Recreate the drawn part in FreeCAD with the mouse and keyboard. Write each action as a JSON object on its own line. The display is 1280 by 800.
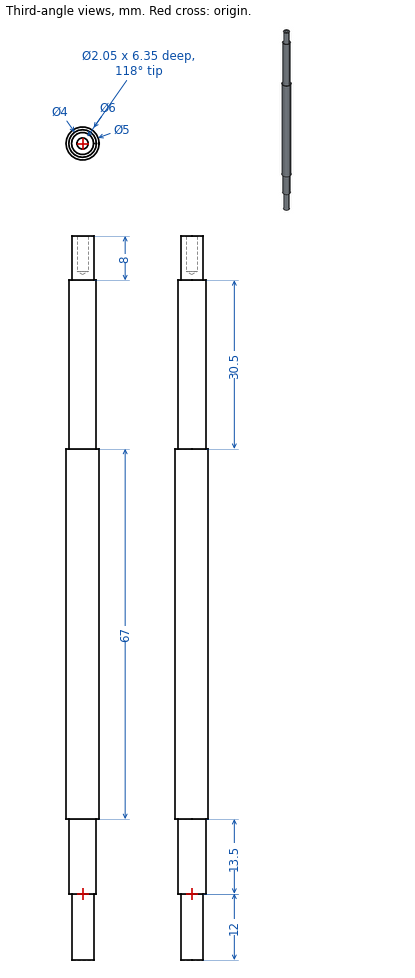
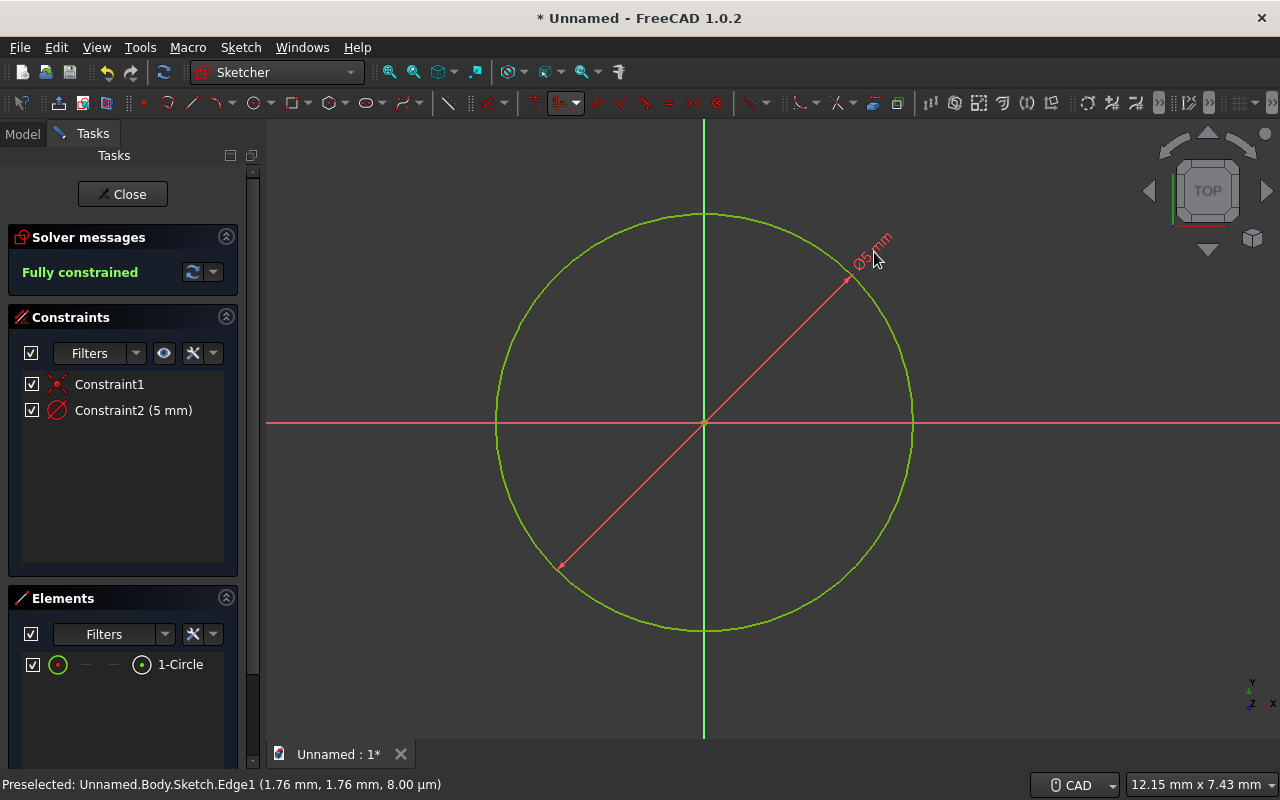
{"action": "left_click", "coordinate": [123, 194]}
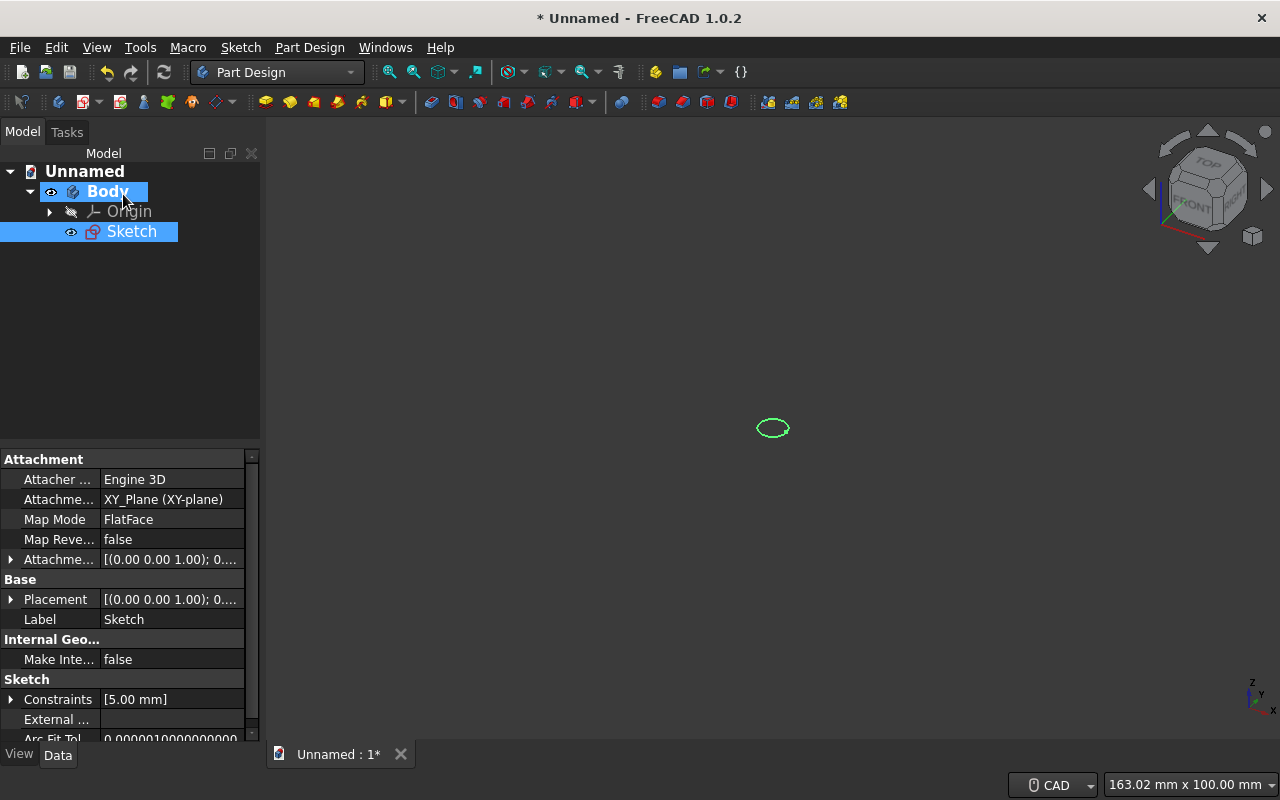
{"action": "left_click", "coordinate": [266, 102]}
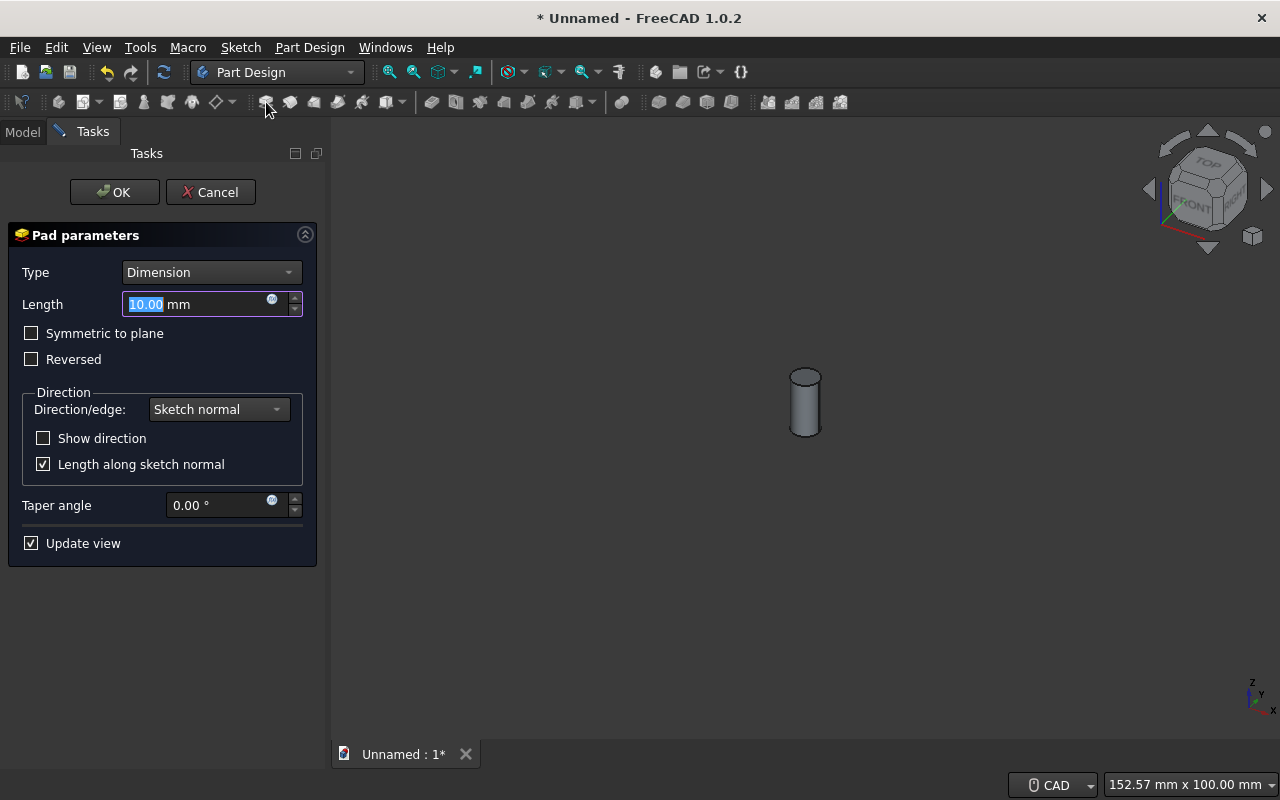
{"action": "type", "text": "13.5"}
{"action": "key", "text": "Tab"}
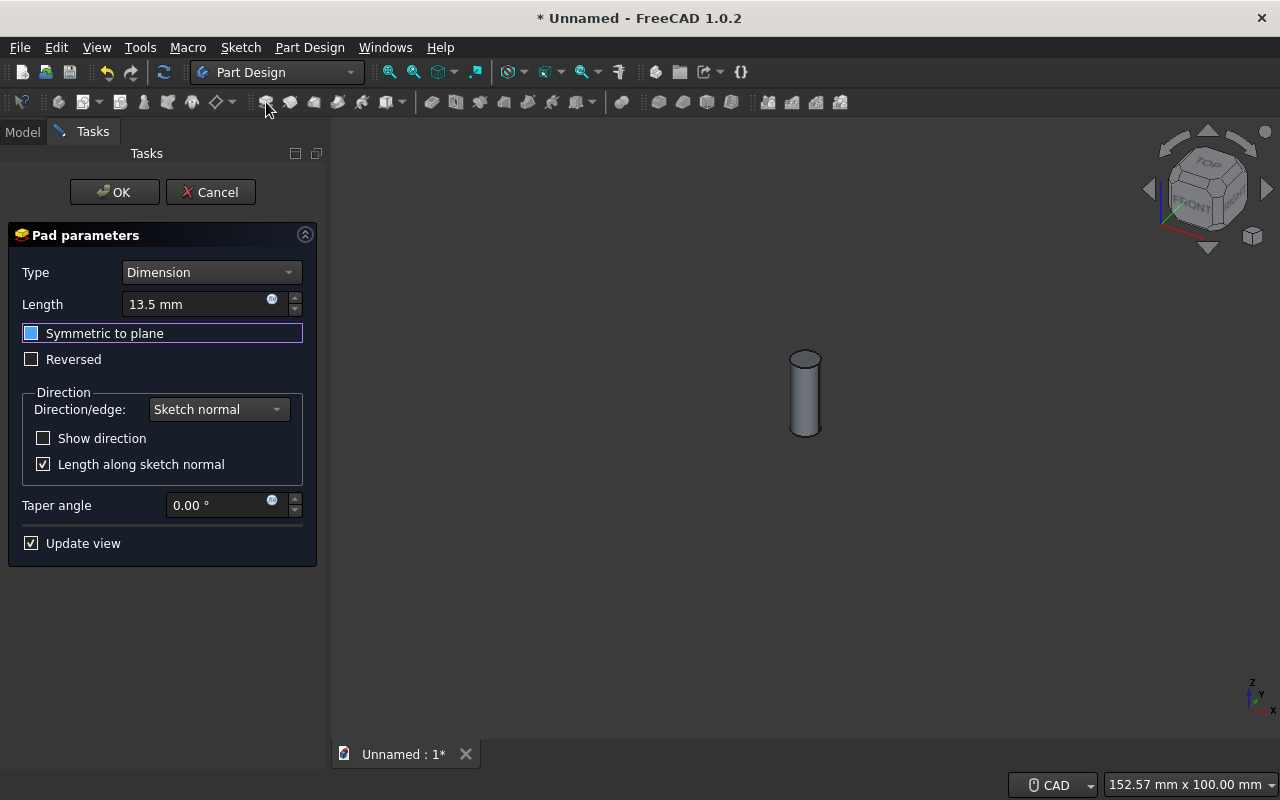
{"action": "left_click", "coordinate": [115, 192]}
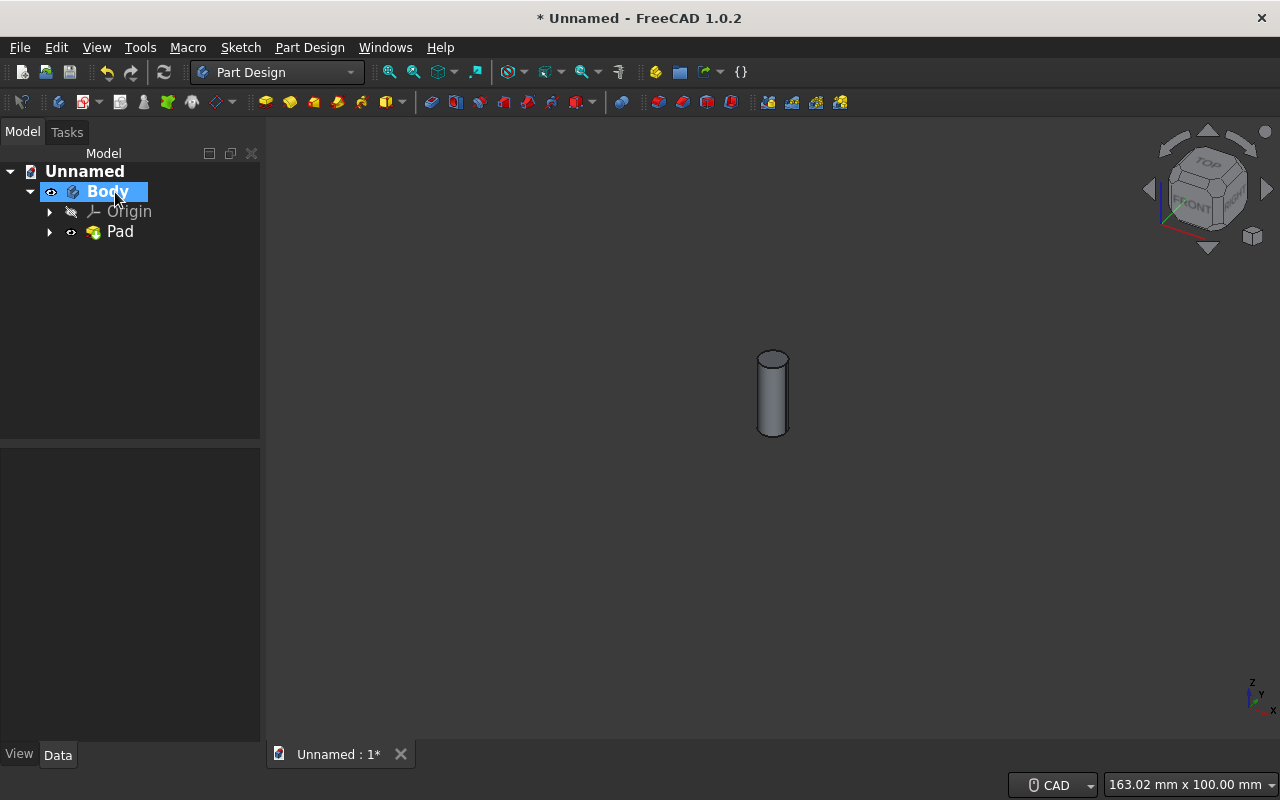
{"action": "left_click", "coordinate": [390, 72]}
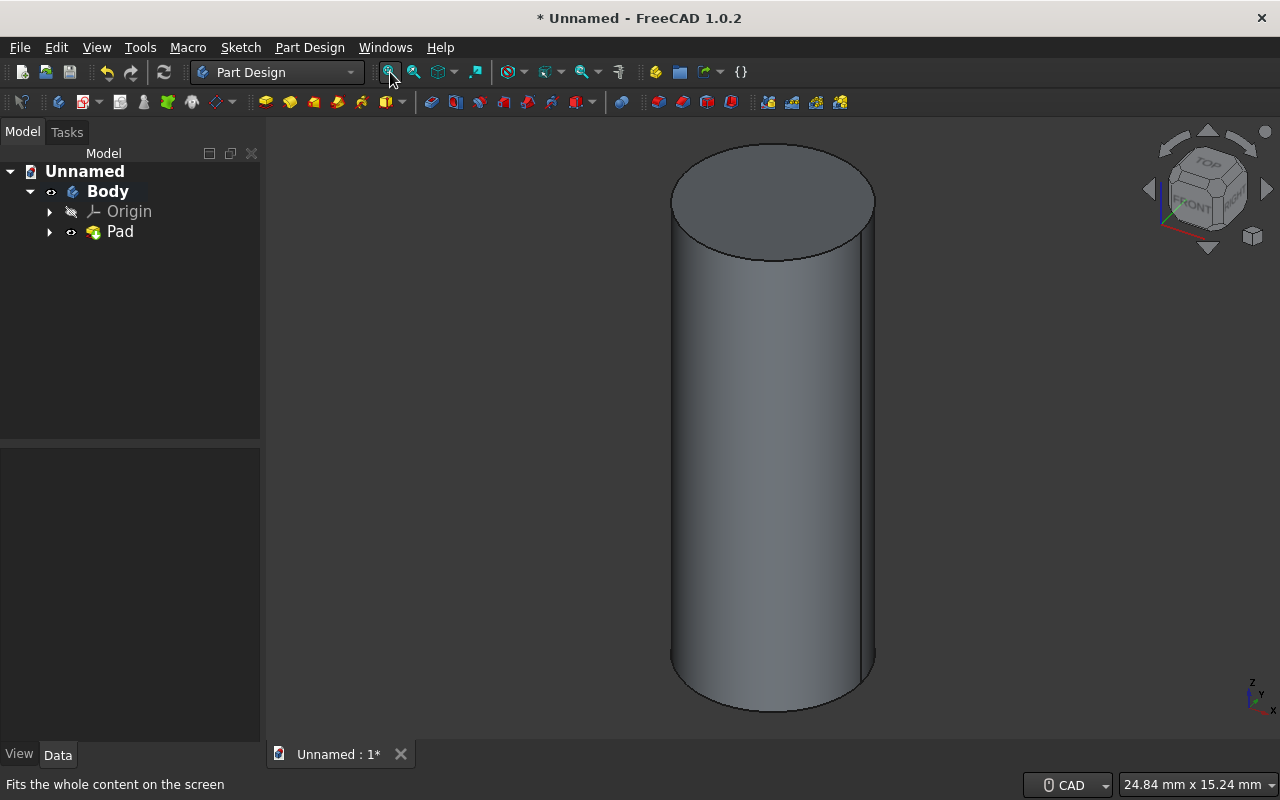
{"action": "left_click", "coordinate": [773, 201]}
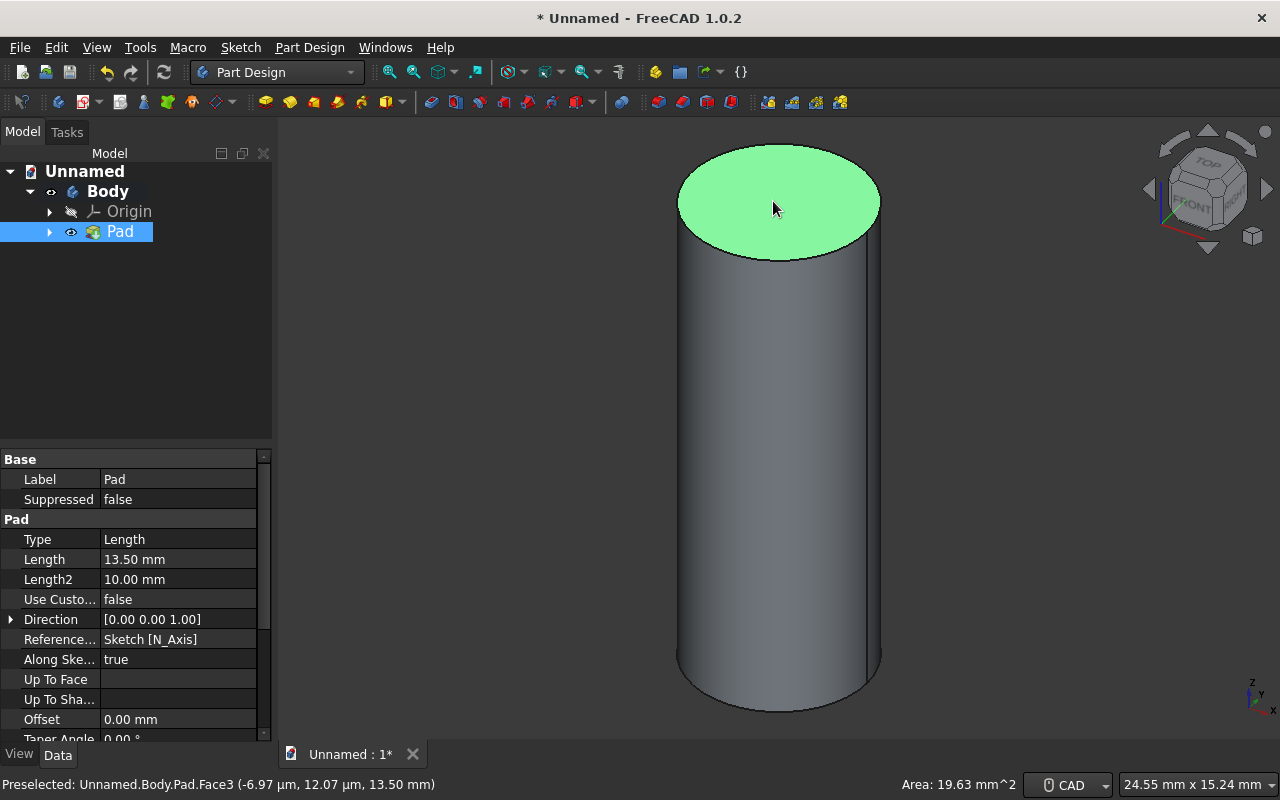
{"action": "left_click", "coordinate": [84, 102]}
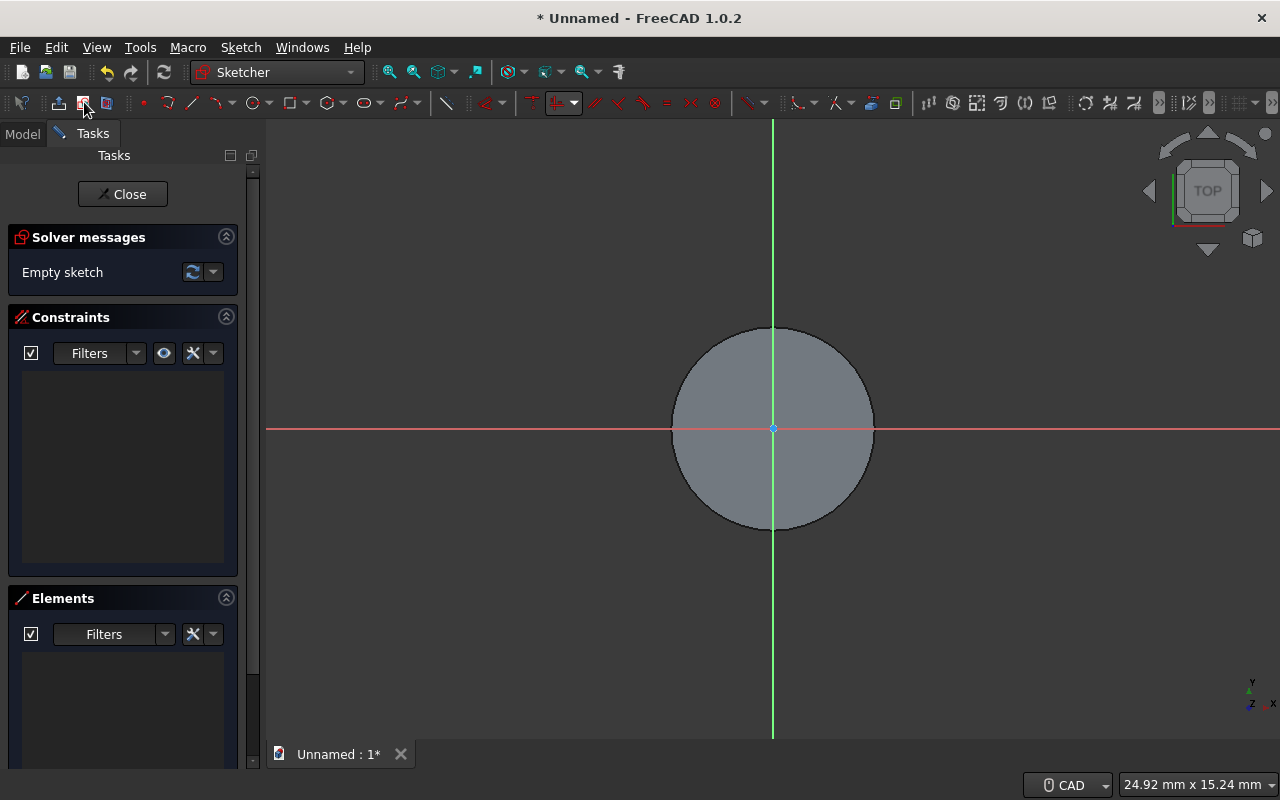
{"action": "scroll", "coordinate": [912, 429], "scroll_direction": "up", "scroll_amount": 2}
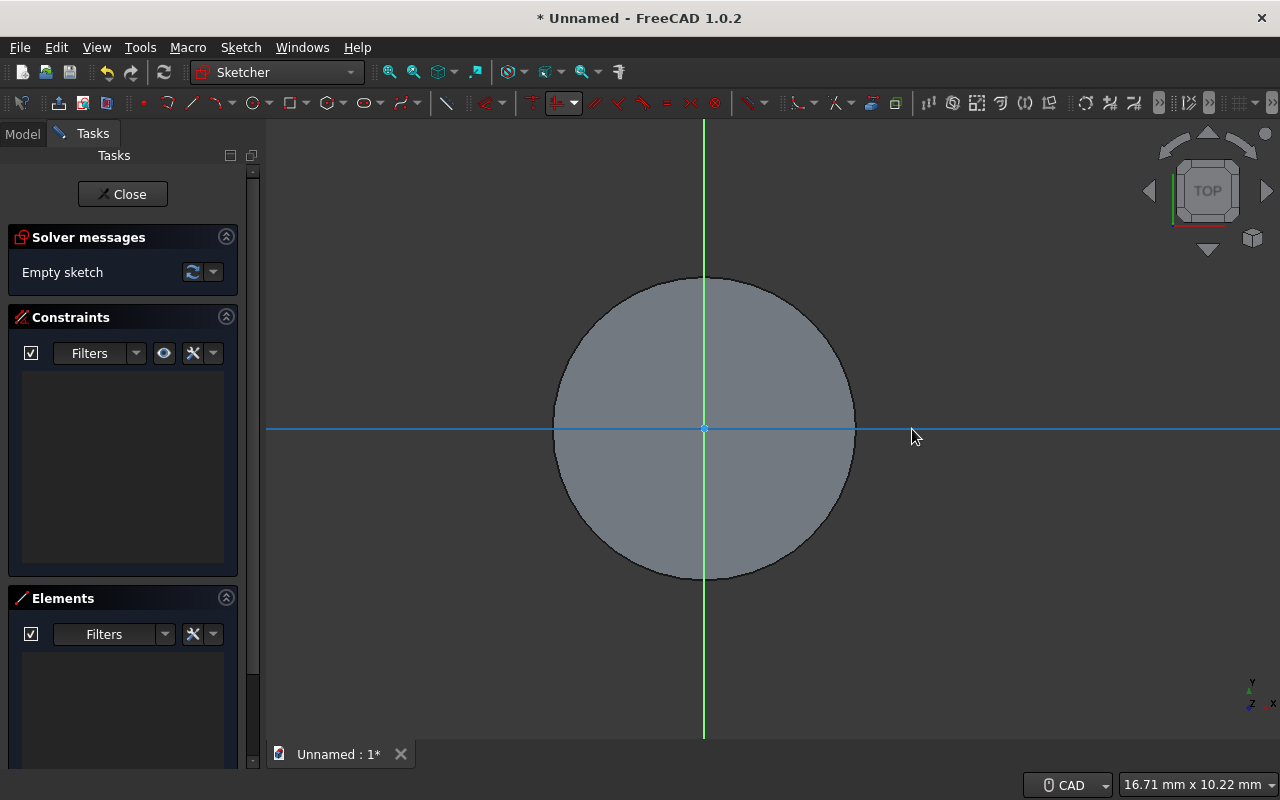
{"action": "left_click", "coordinate": [254, 104]}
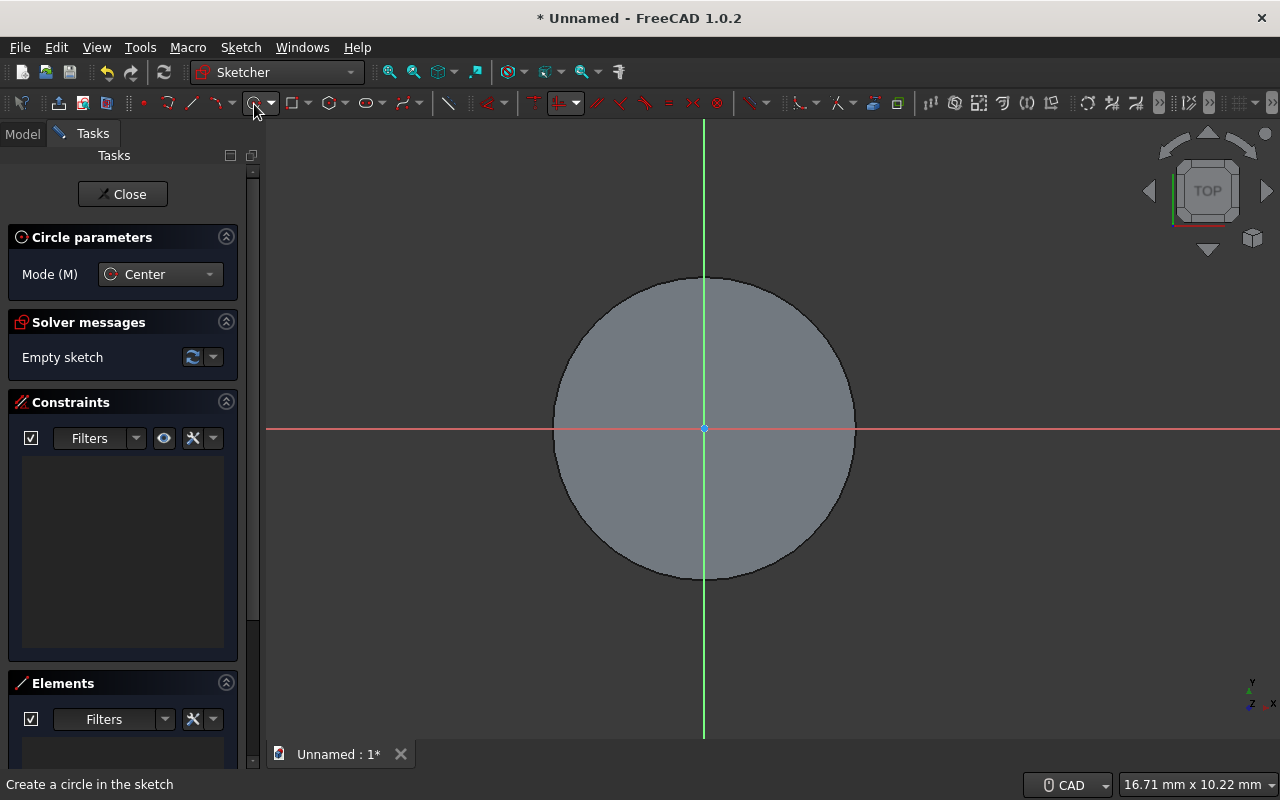
{"action": "left_click", "coordinate": [704, 429]}
{"action": "left_click", "coordinate": [833, 300]}
{"action": "key", "text": "Escape"}